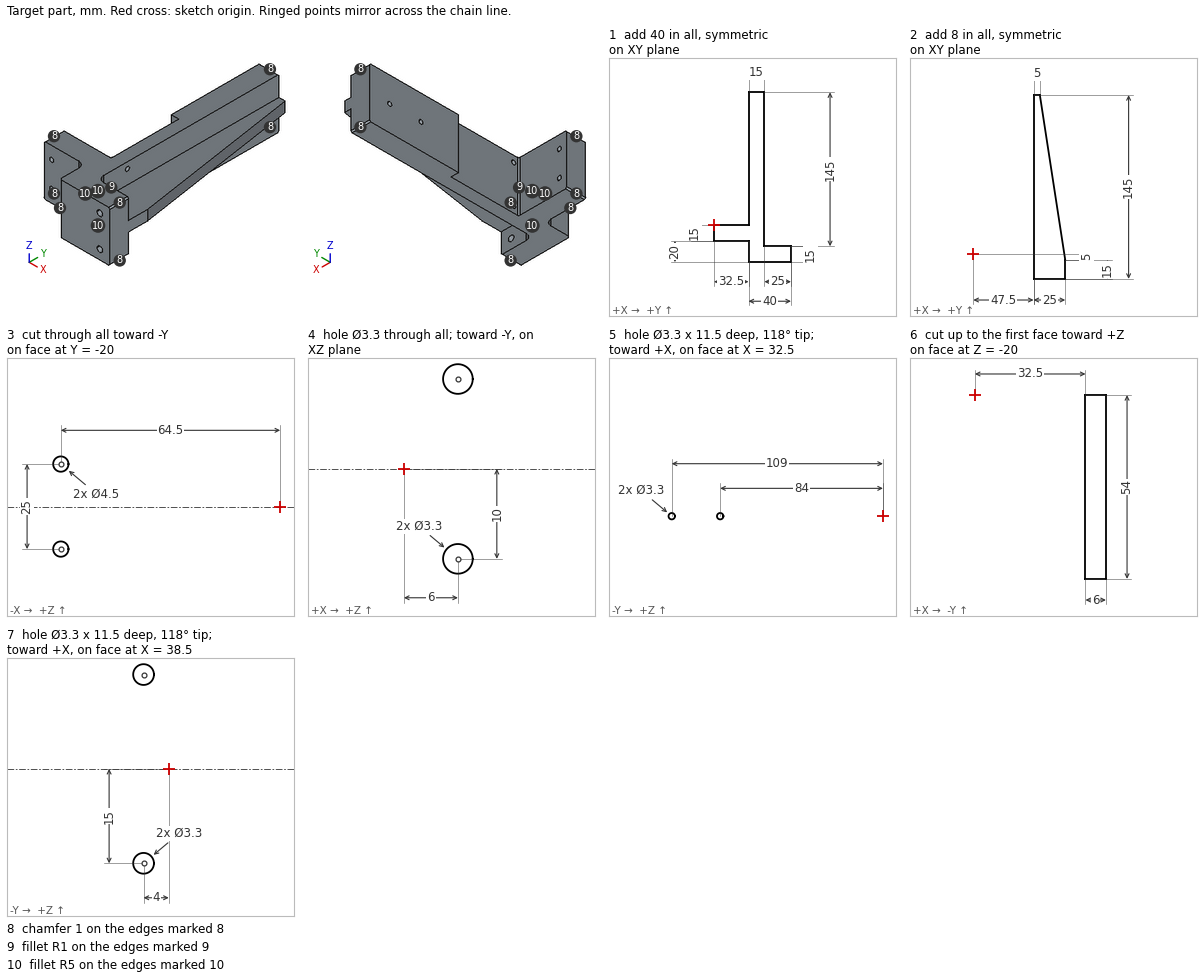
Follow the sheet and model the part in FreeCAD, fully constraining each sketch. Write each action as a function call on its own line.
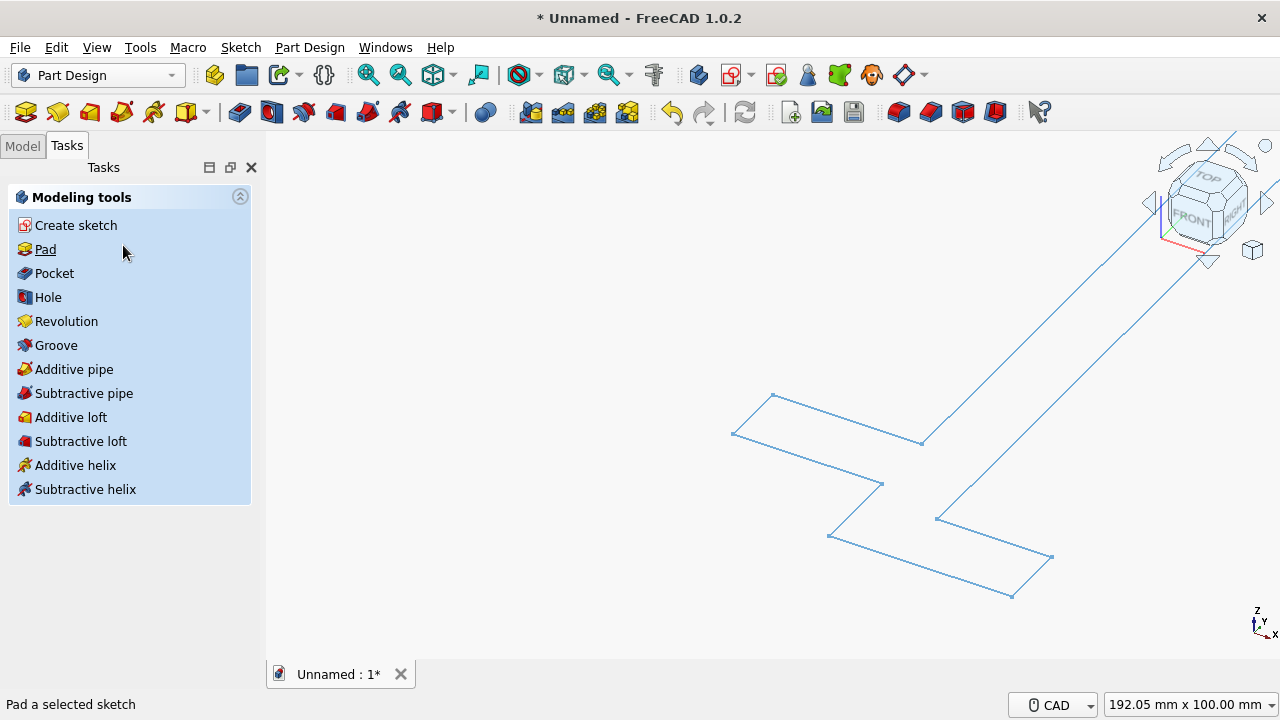
click(26, 112)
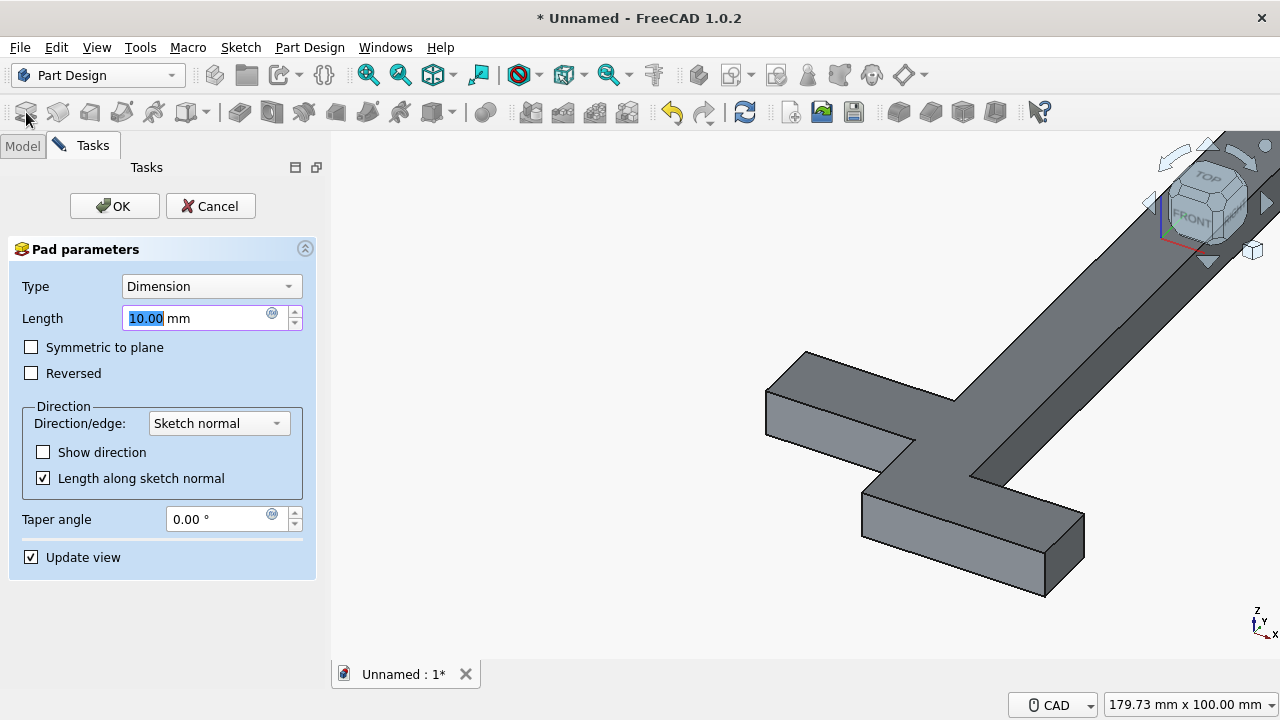
text(40)
key(Tab)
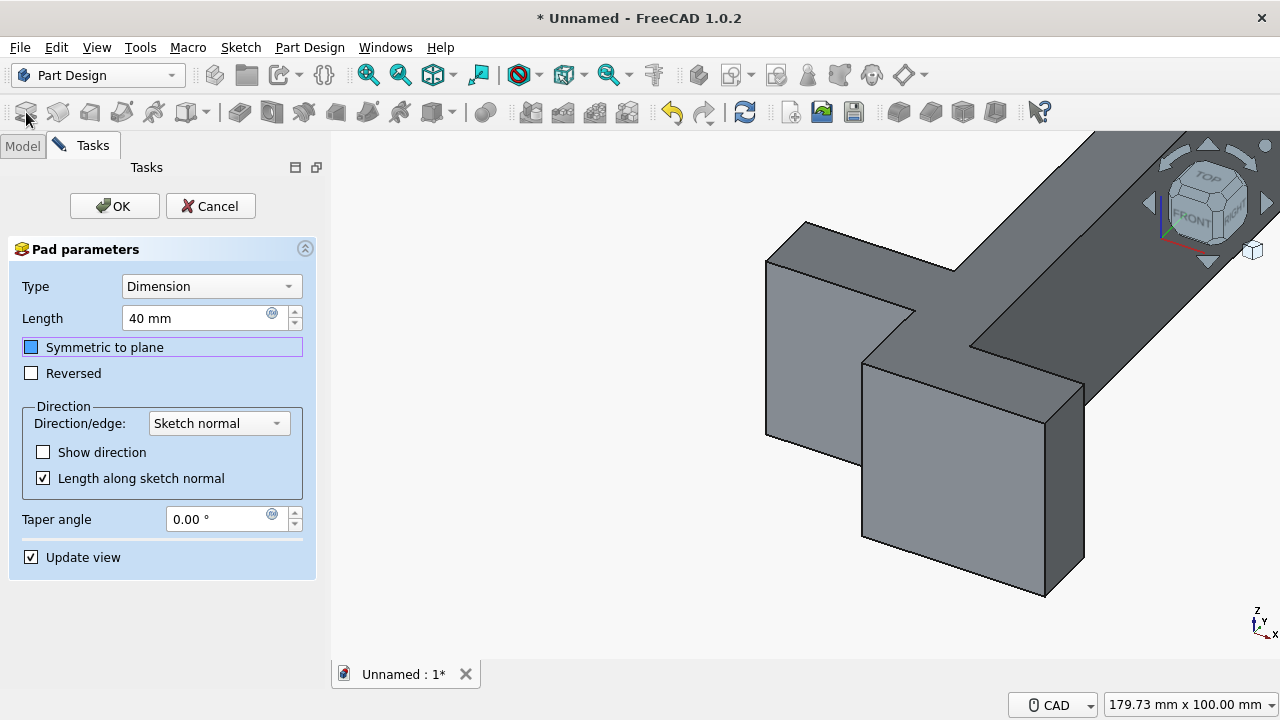
click(30, 347)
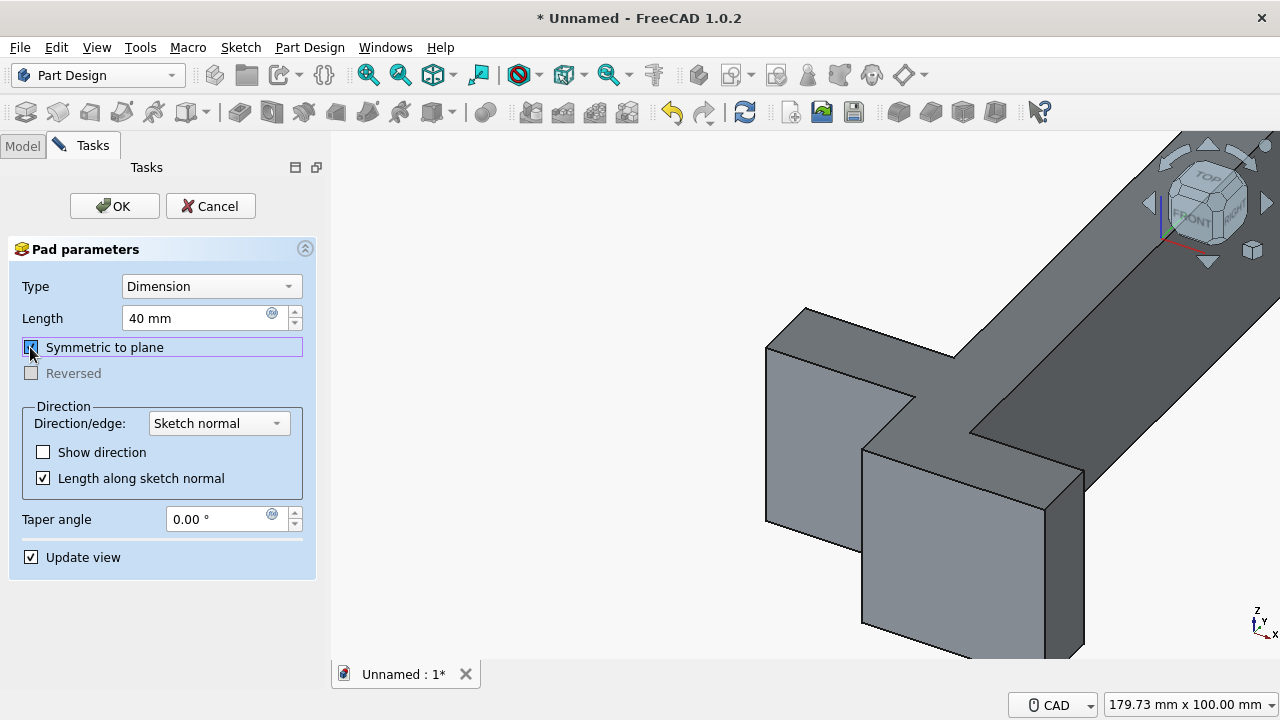
click(115, 206)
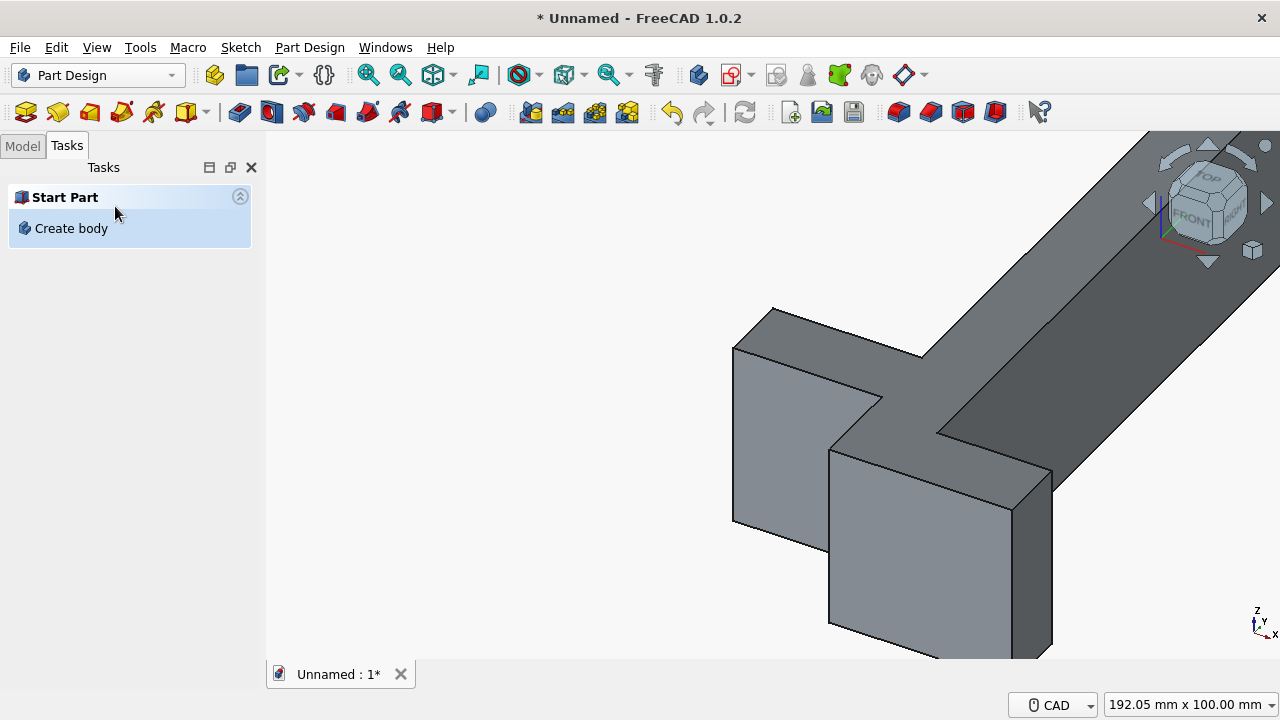
click(370, 76)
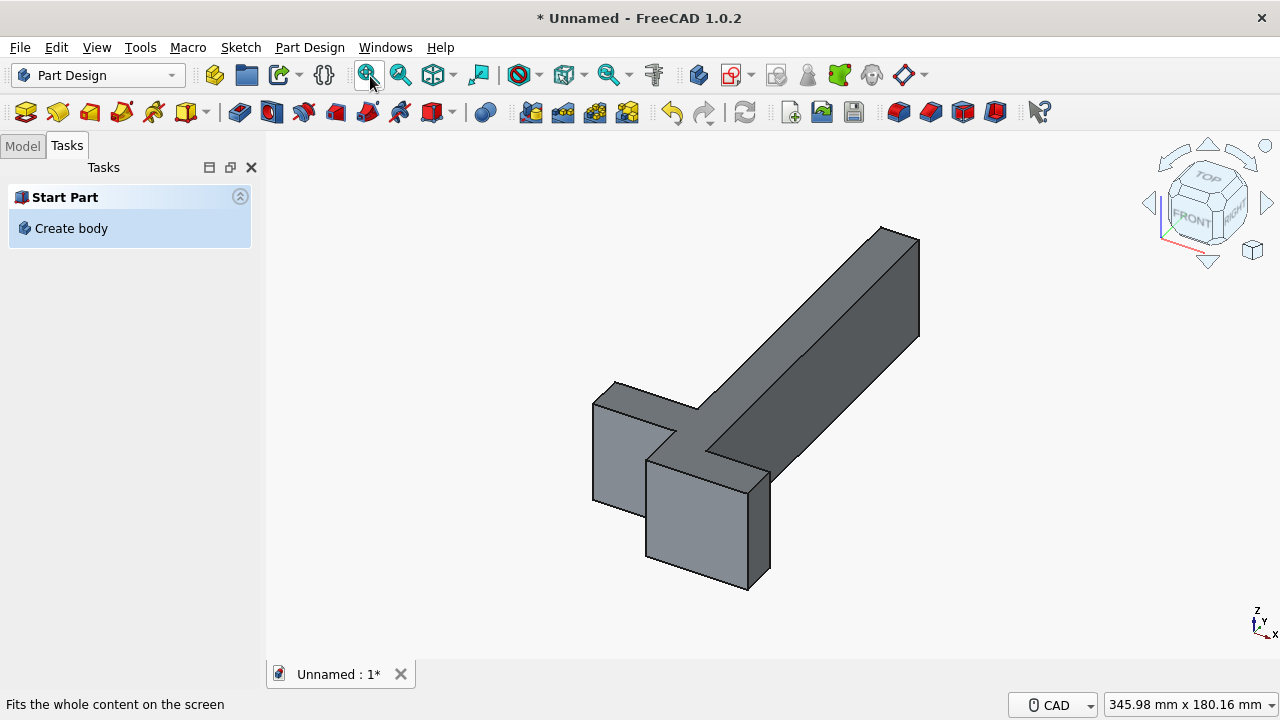
click(732, 76)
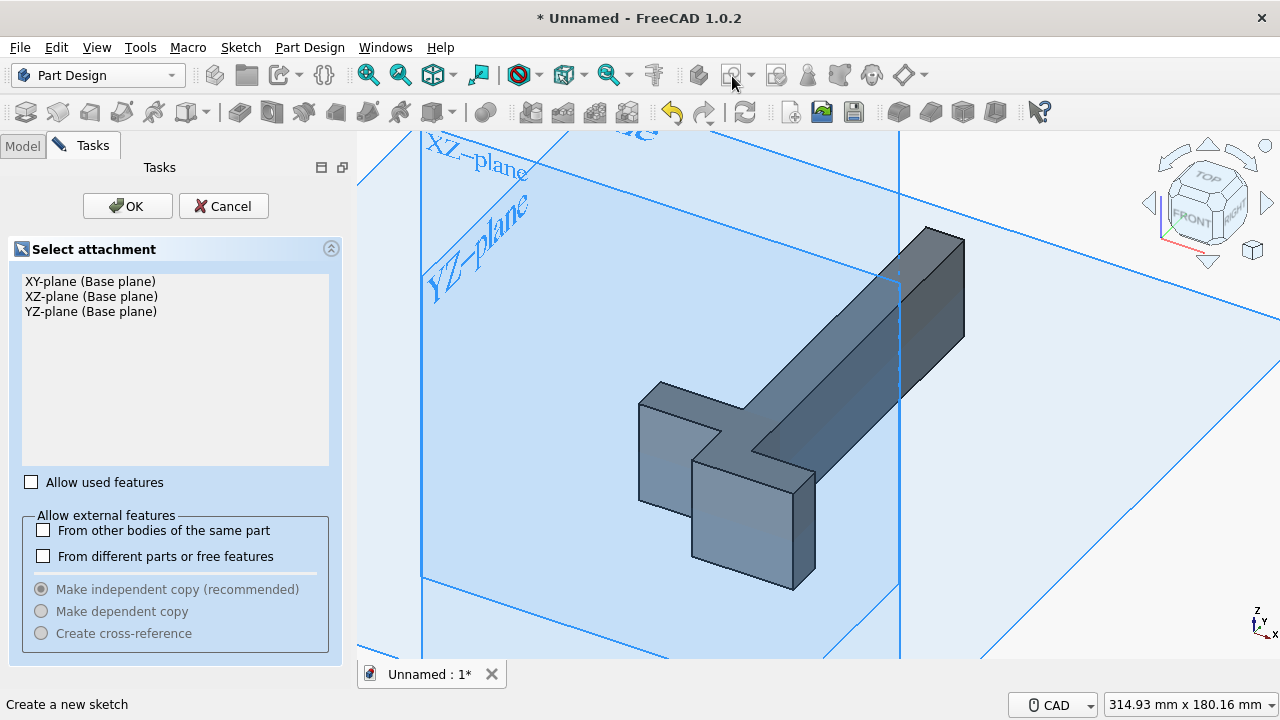
click(82, 282)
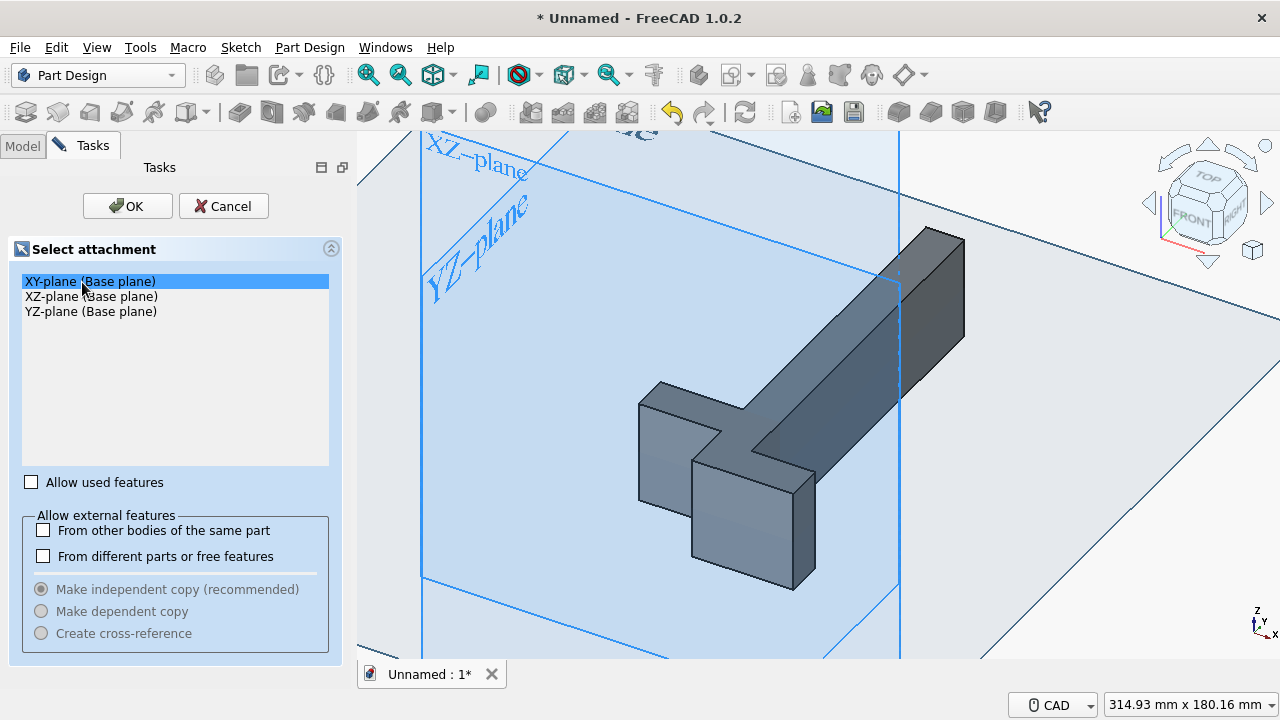
click(128, 206)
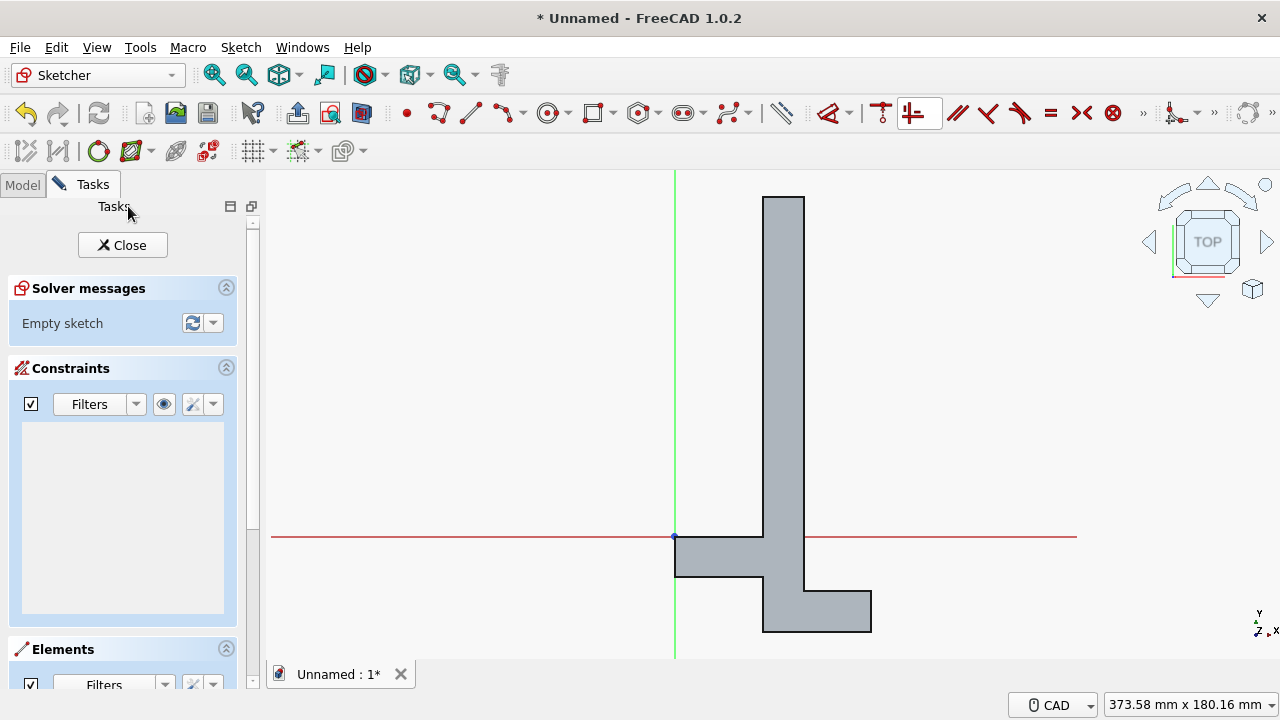
click(362, 114)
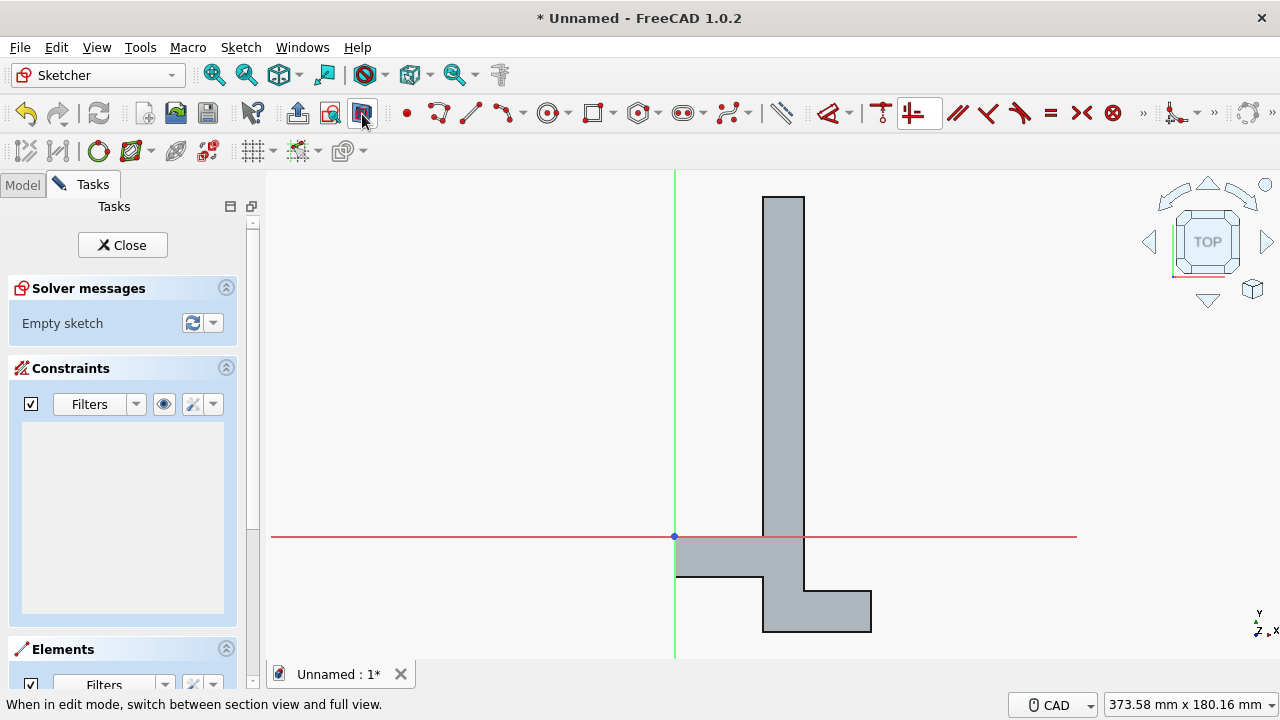
scroll(395, 506, down, 1)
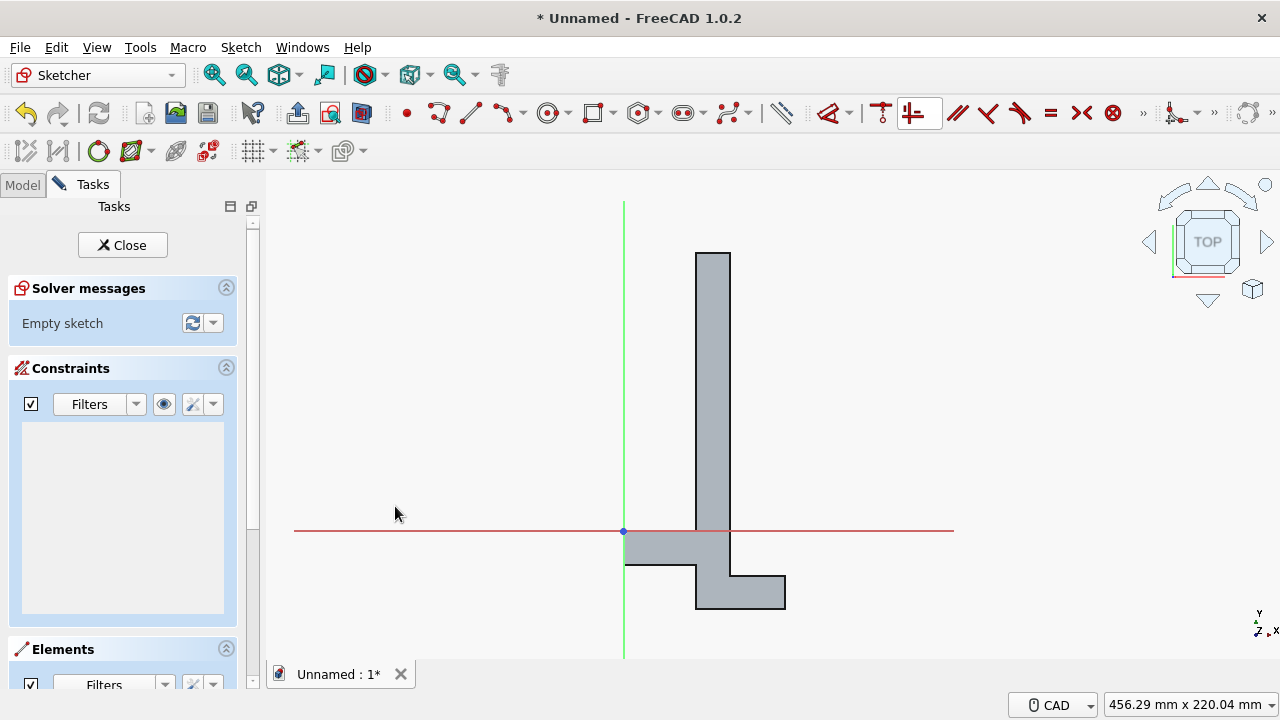
key(g)
key(m)